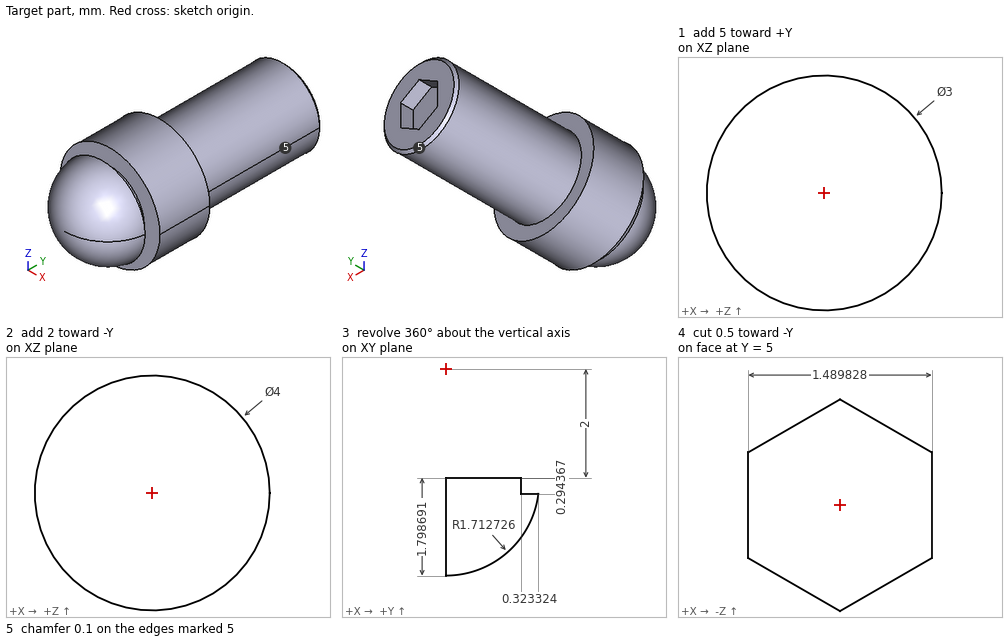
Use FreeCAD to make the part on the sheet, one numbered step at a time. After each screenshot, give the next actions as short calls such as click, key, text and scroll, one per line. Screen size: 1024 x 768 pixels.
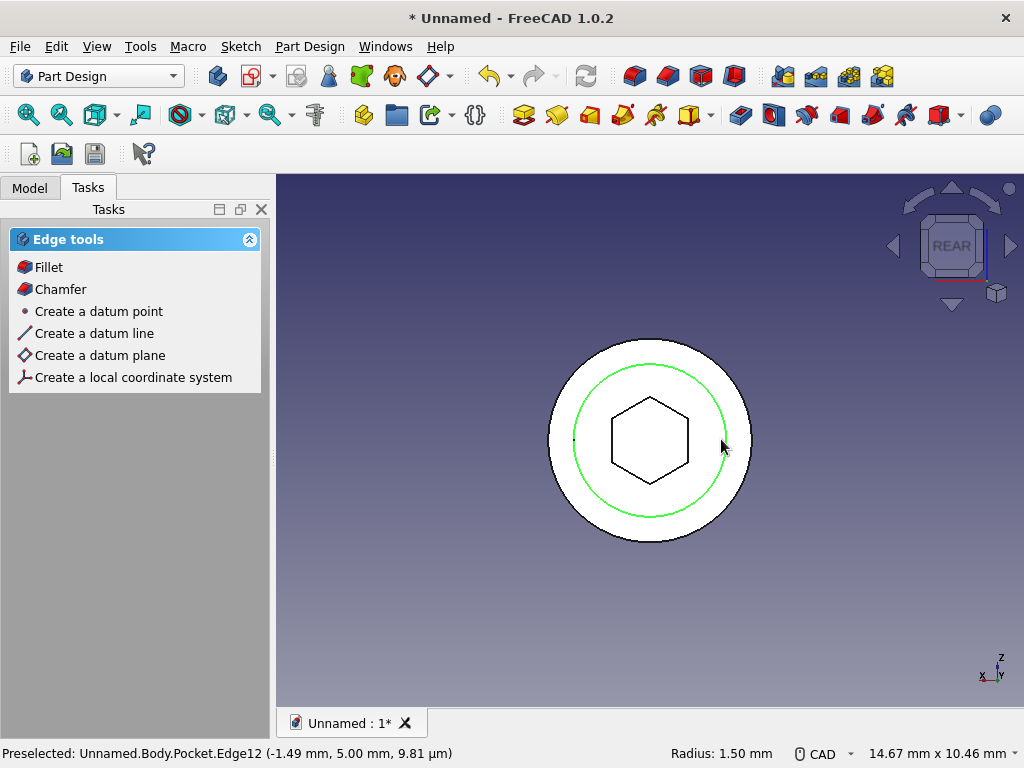
click(668, 76)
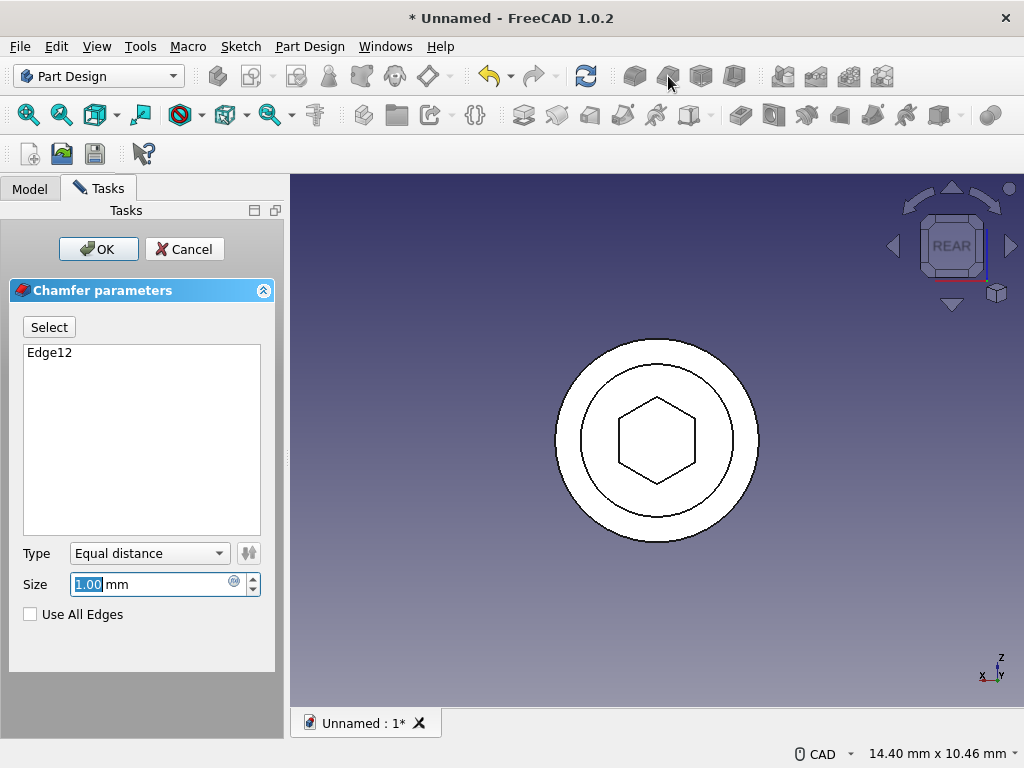
text(0.1)
key(Tab)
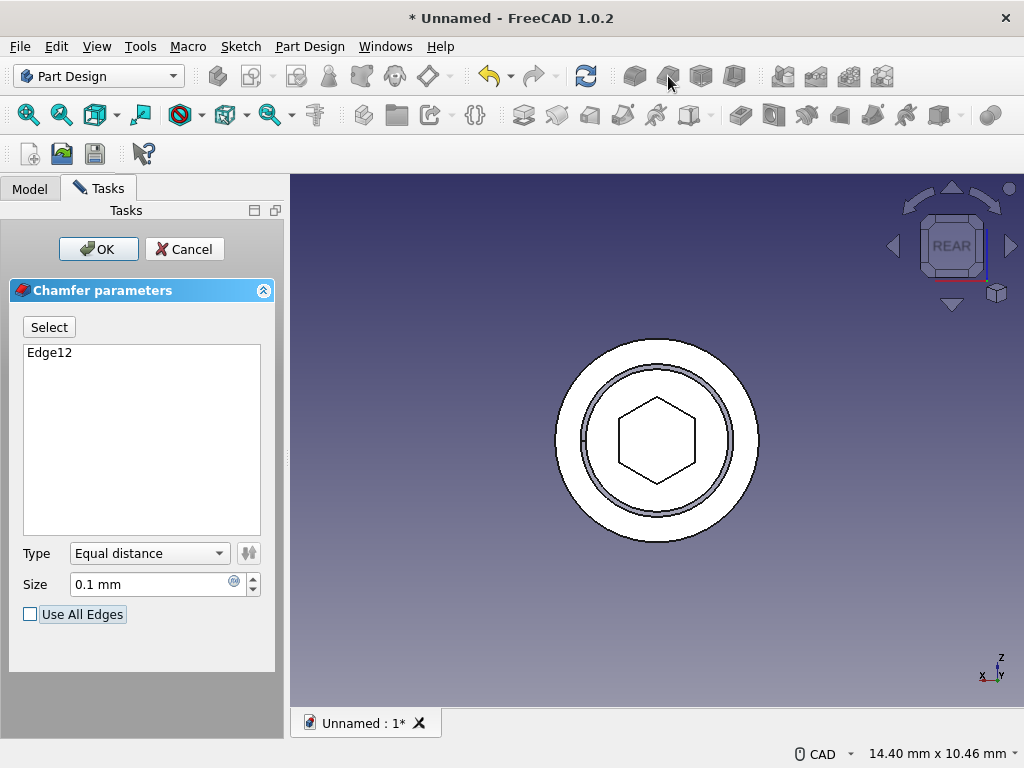
click(99, 249)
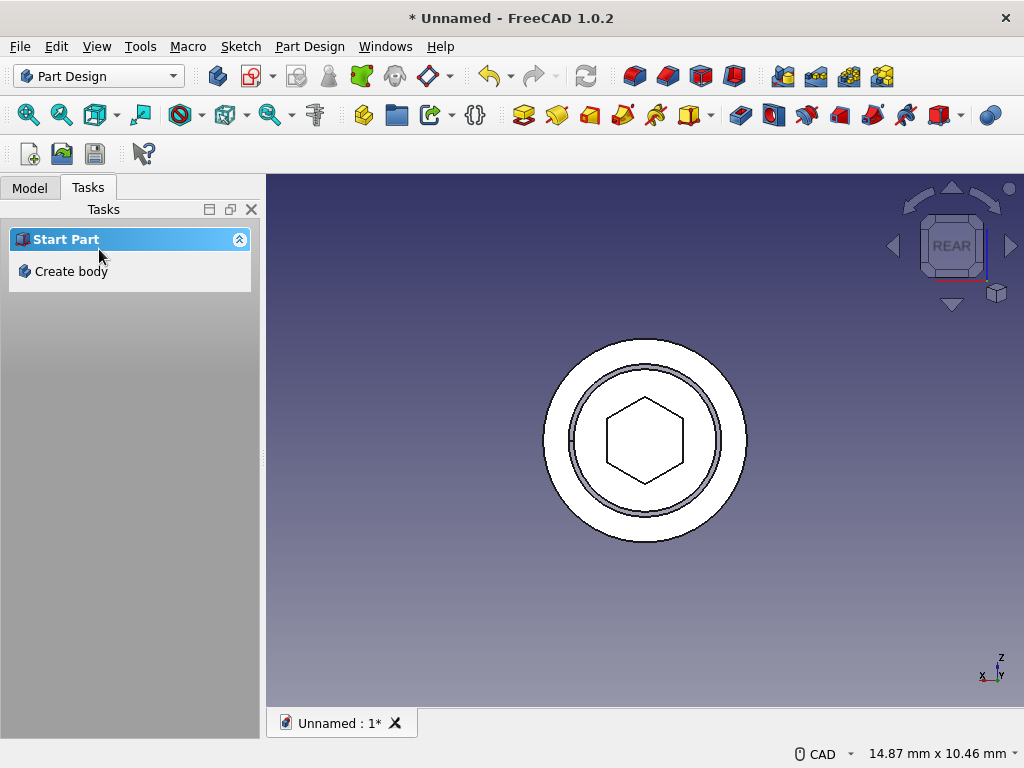
key(0)